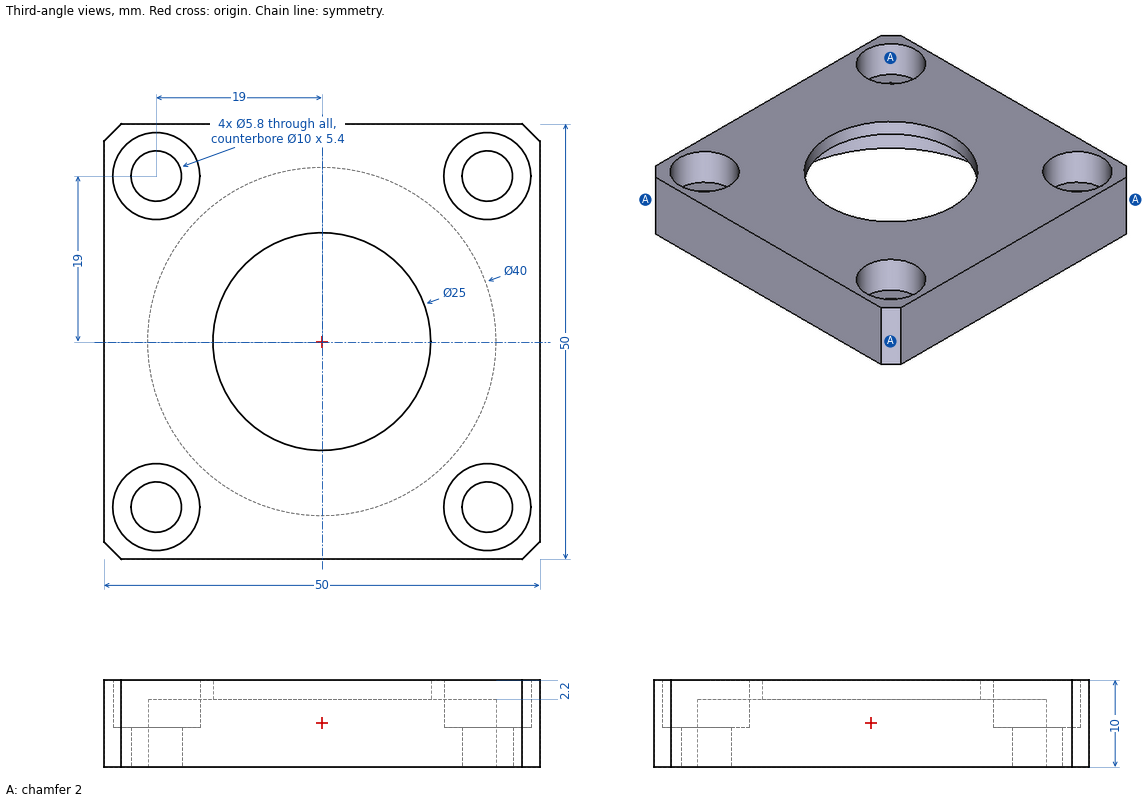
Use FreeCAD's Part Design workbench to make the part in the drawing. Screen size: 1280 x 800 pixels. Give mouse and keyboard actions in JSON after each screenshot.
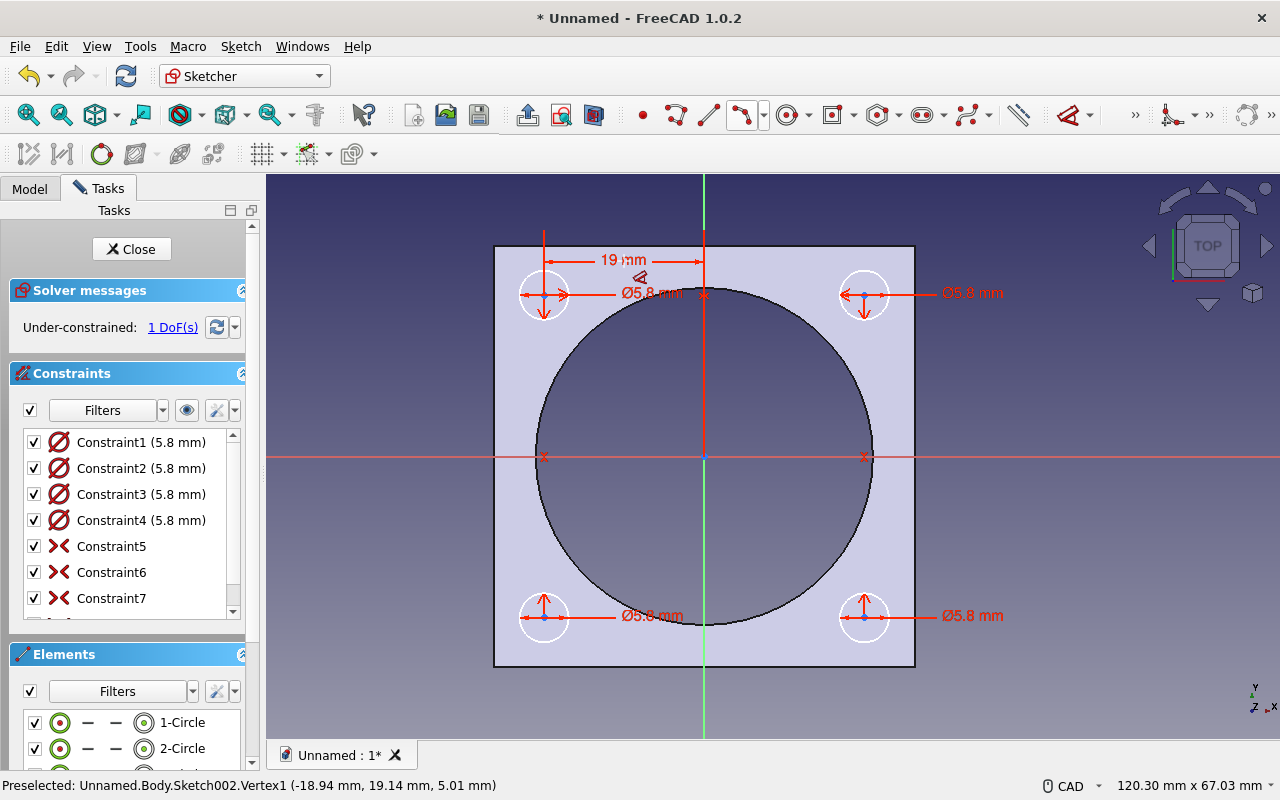
{"action": "left_click", "coordinate": [544, 295]}
{"action": "left_click", "coordinate": [510, 376]}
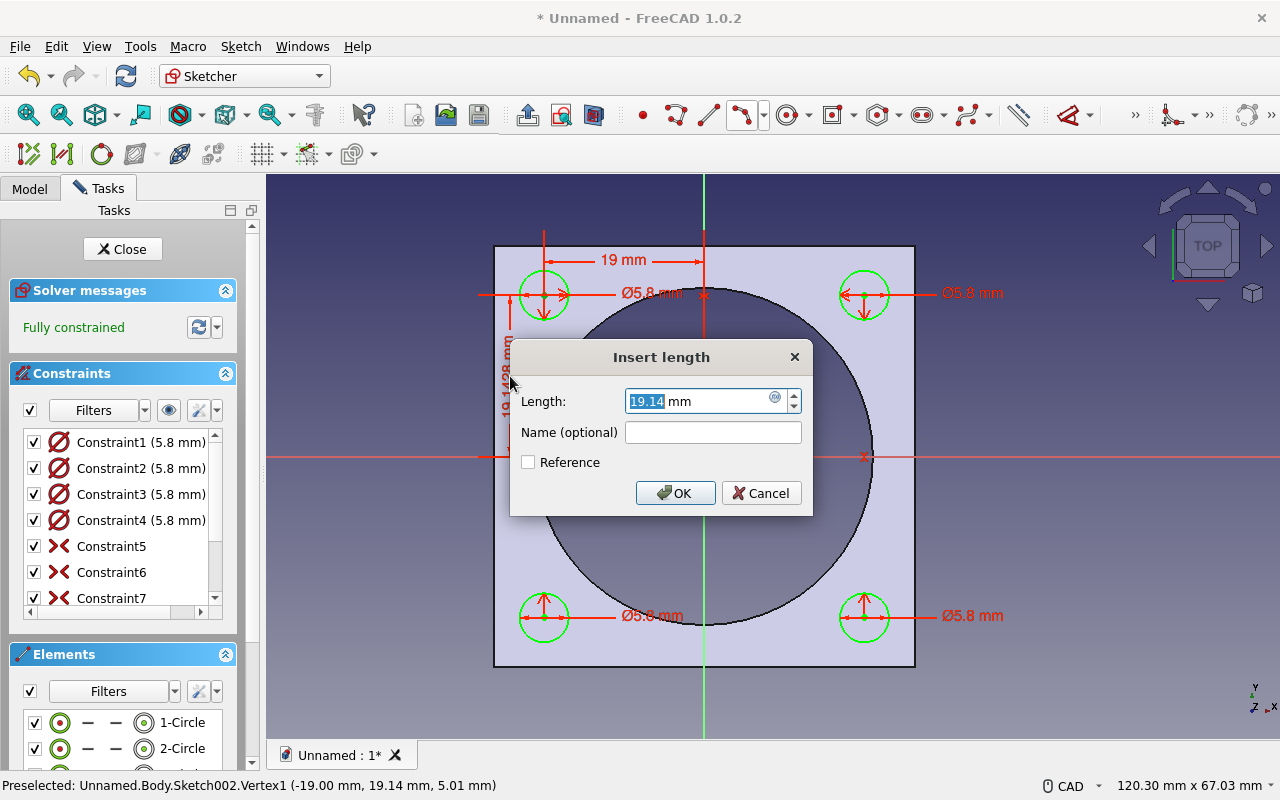
{"action": "type", "text": "19"}
{"action": "key", "text": "Return"}
{"action": "key", "text": "Escape"}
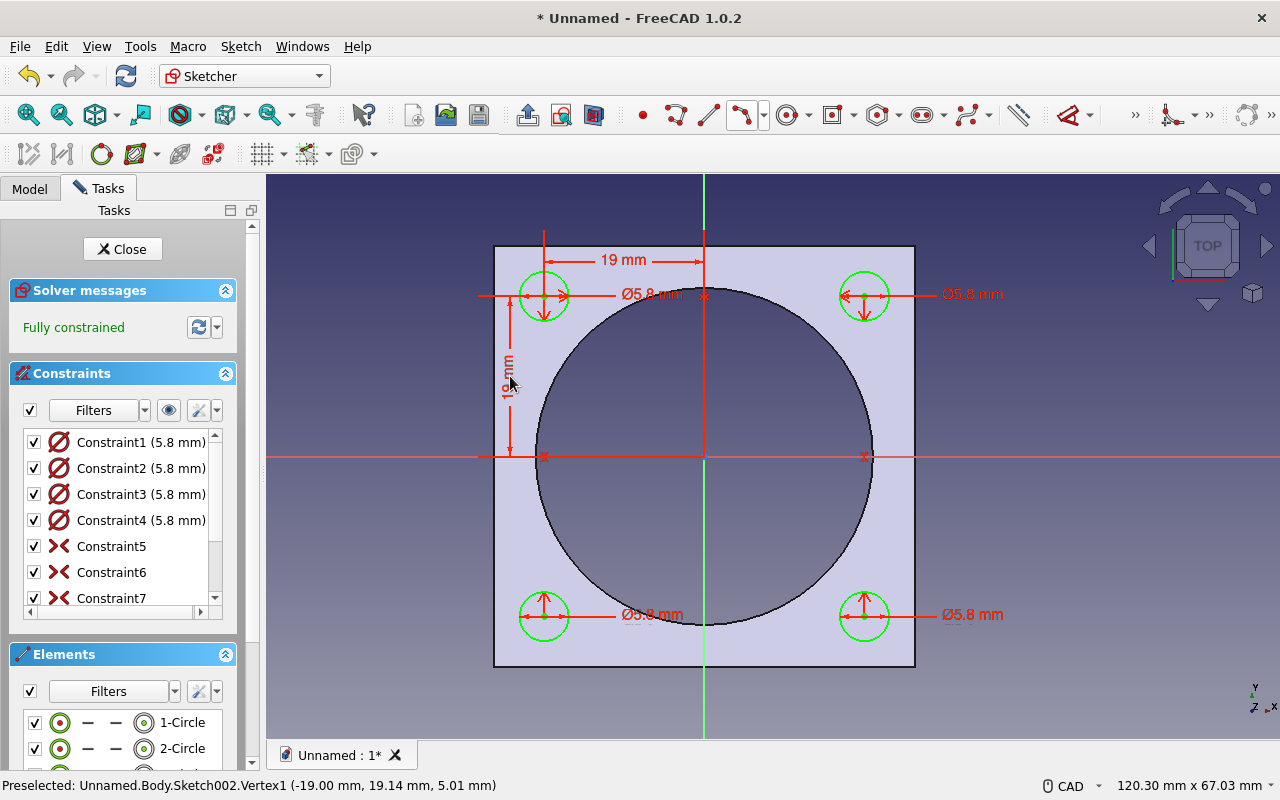
{"action": "left_click", "coordinate": [123, 249]}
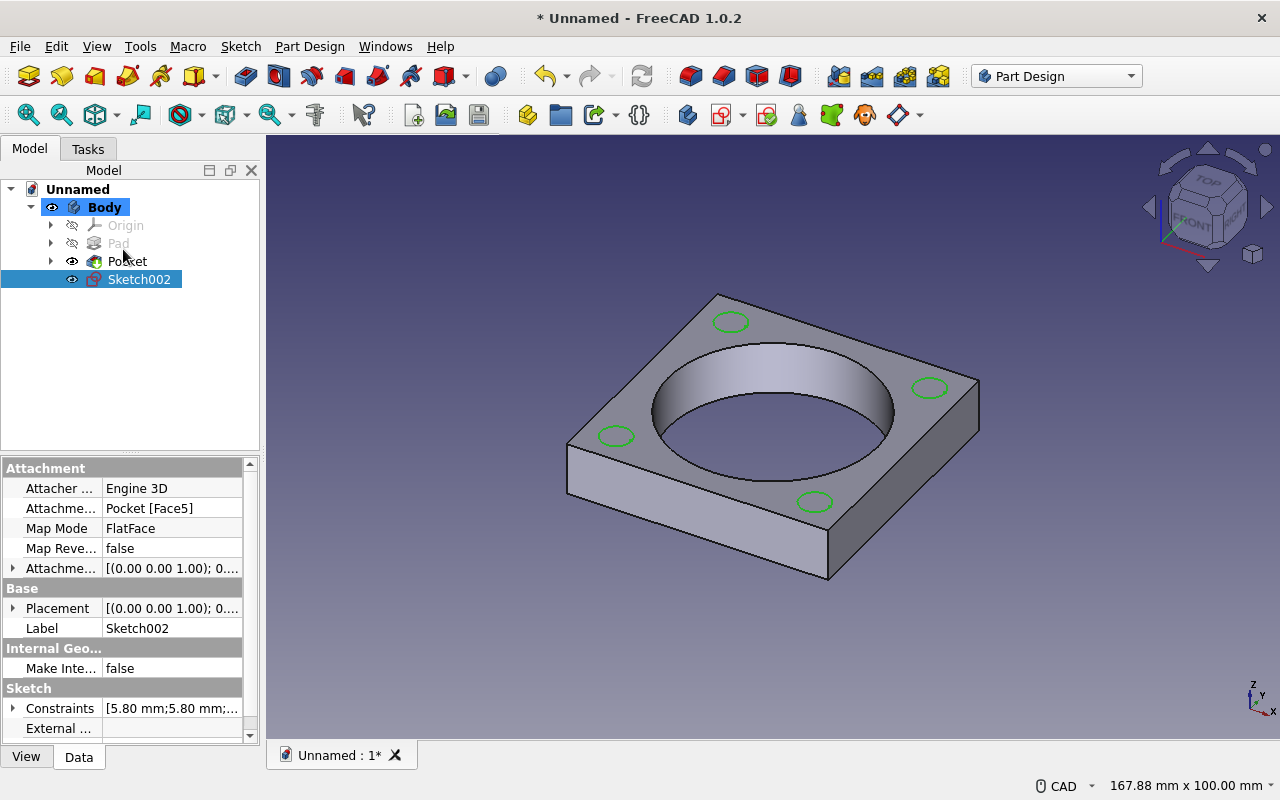
{"action": "left_click", "coordinate": [279, 76]}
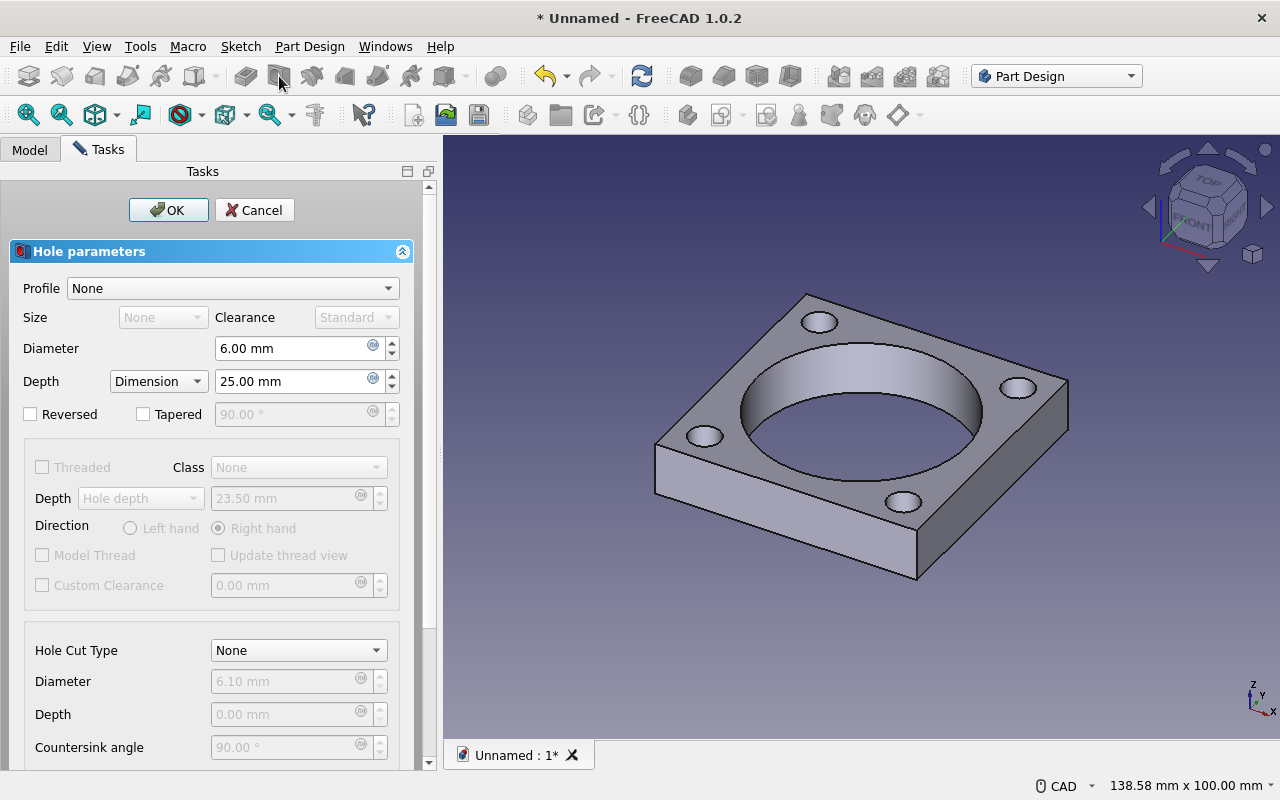
{"action": "triple_click", "coordinate": [300, 348]}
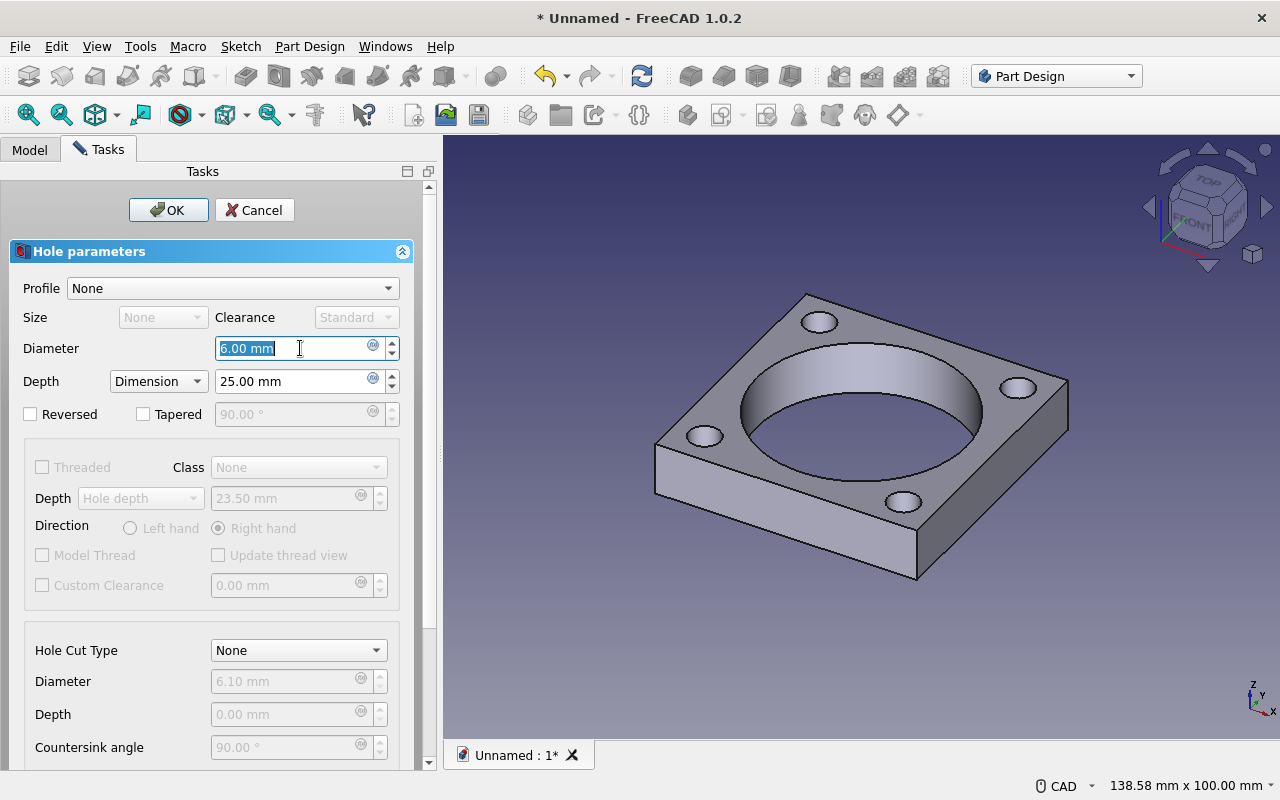
{"action": "type", "text": "5.8"}
{"action": "key", "text": "Tab"}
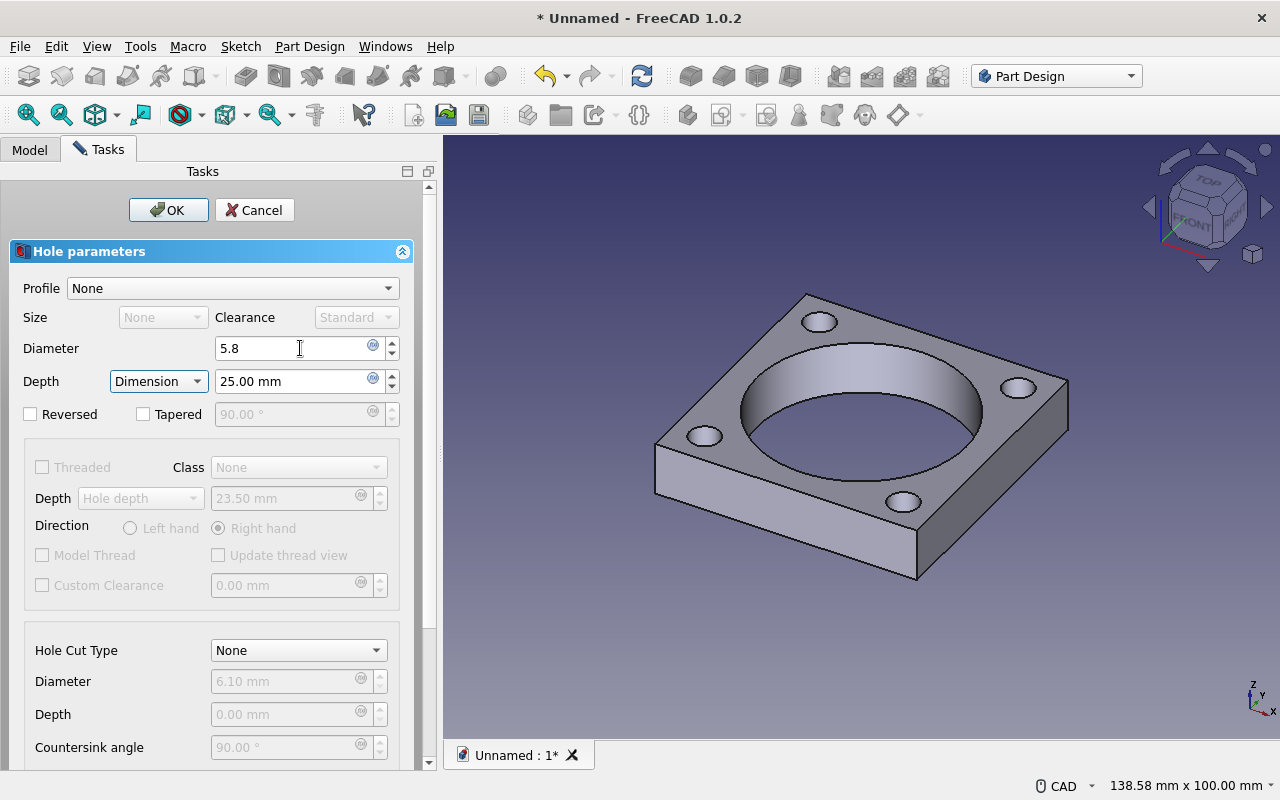
{"action": "left_click", "coordinate": [160, 382]}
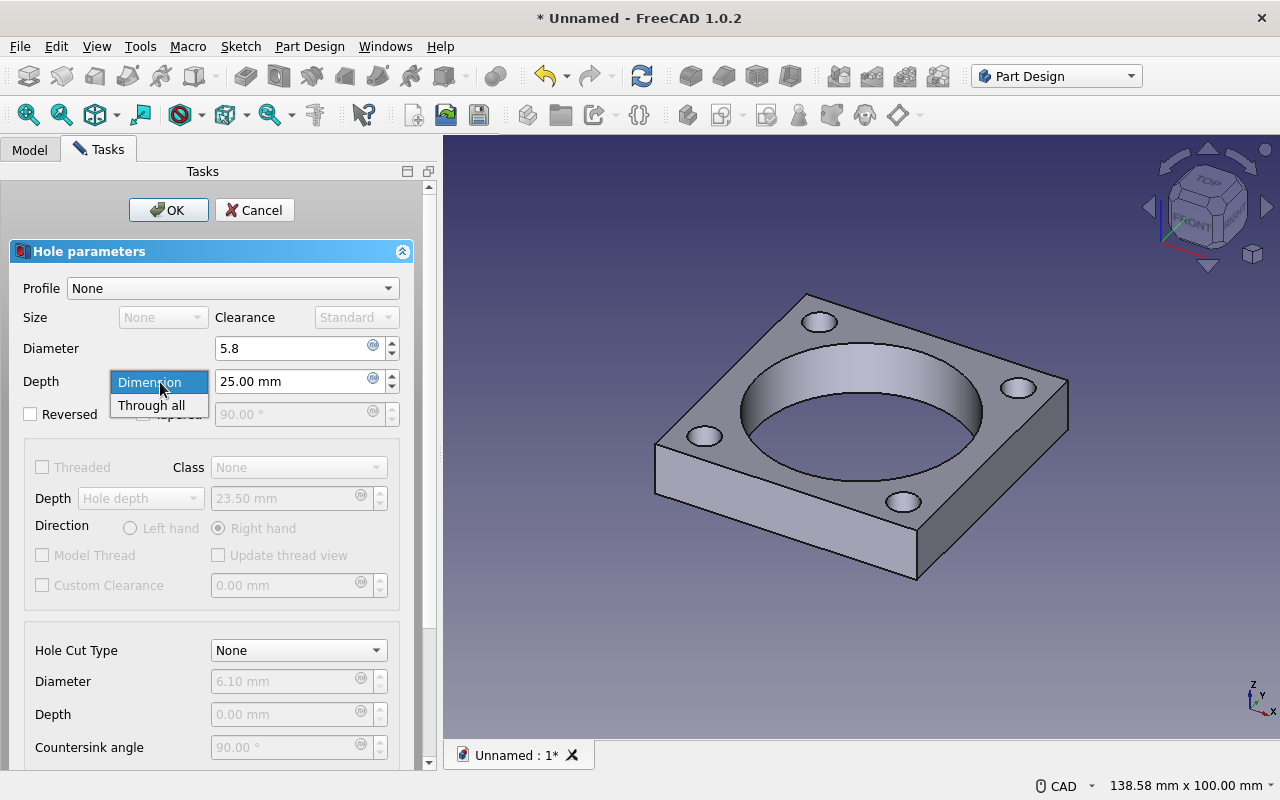
{"action": "left_click", "coordinate": [158, 406]}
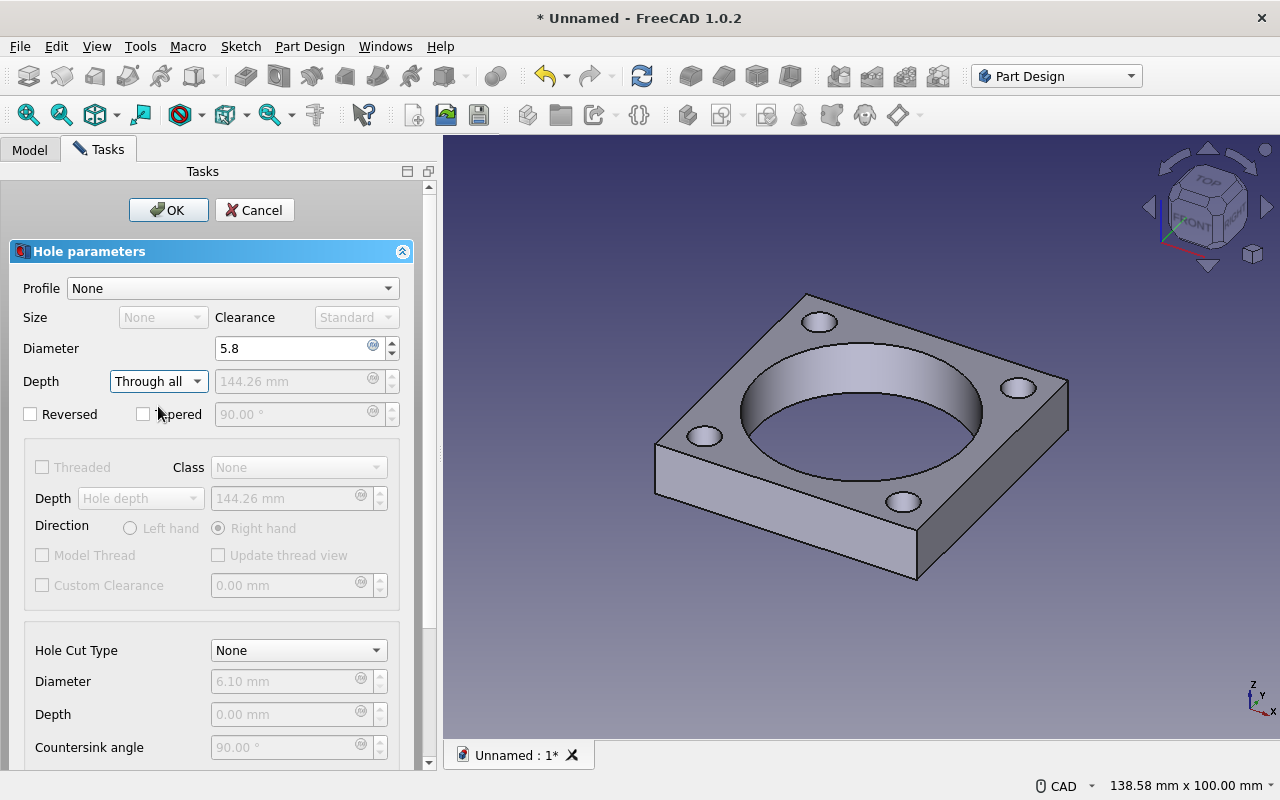
{"action": "left_click", "coordinate": [300, 650]}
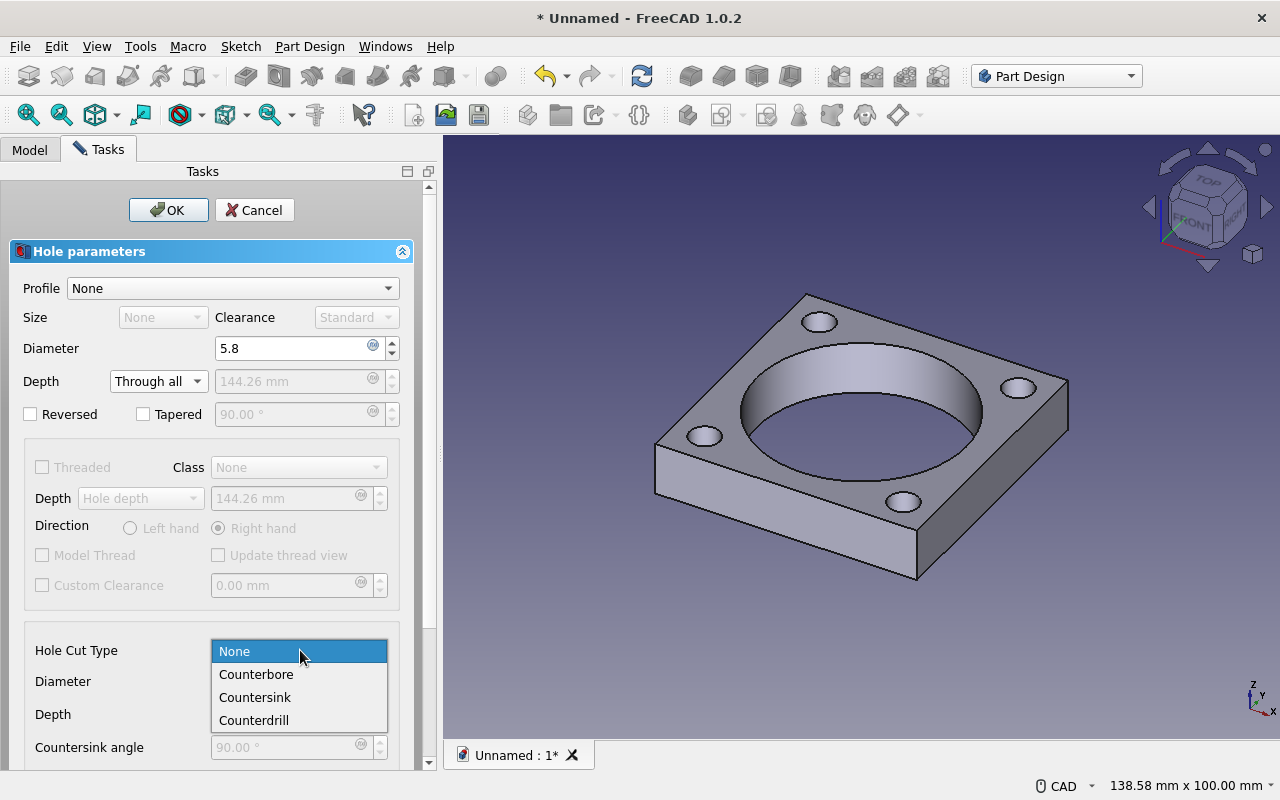
{"action": "left_click", "coordinate": [298, 674]}